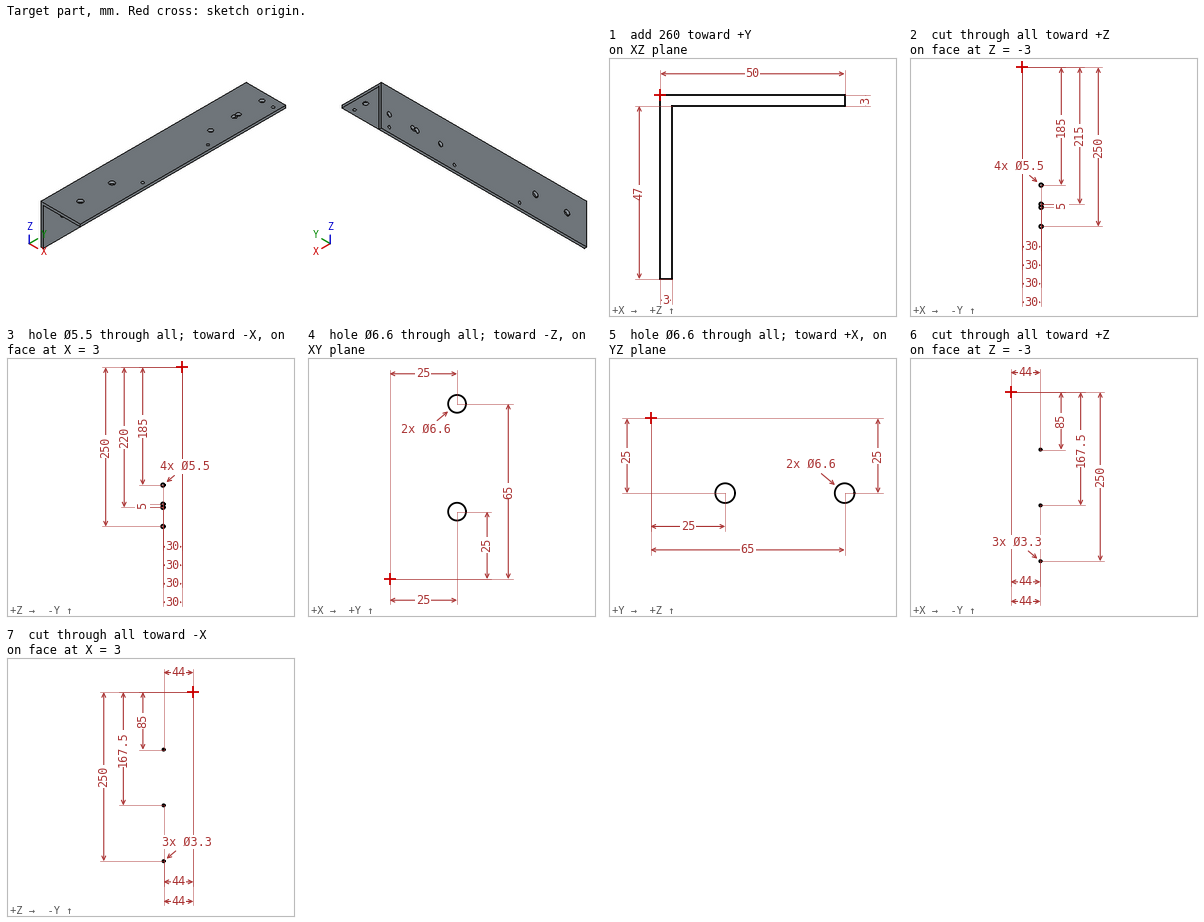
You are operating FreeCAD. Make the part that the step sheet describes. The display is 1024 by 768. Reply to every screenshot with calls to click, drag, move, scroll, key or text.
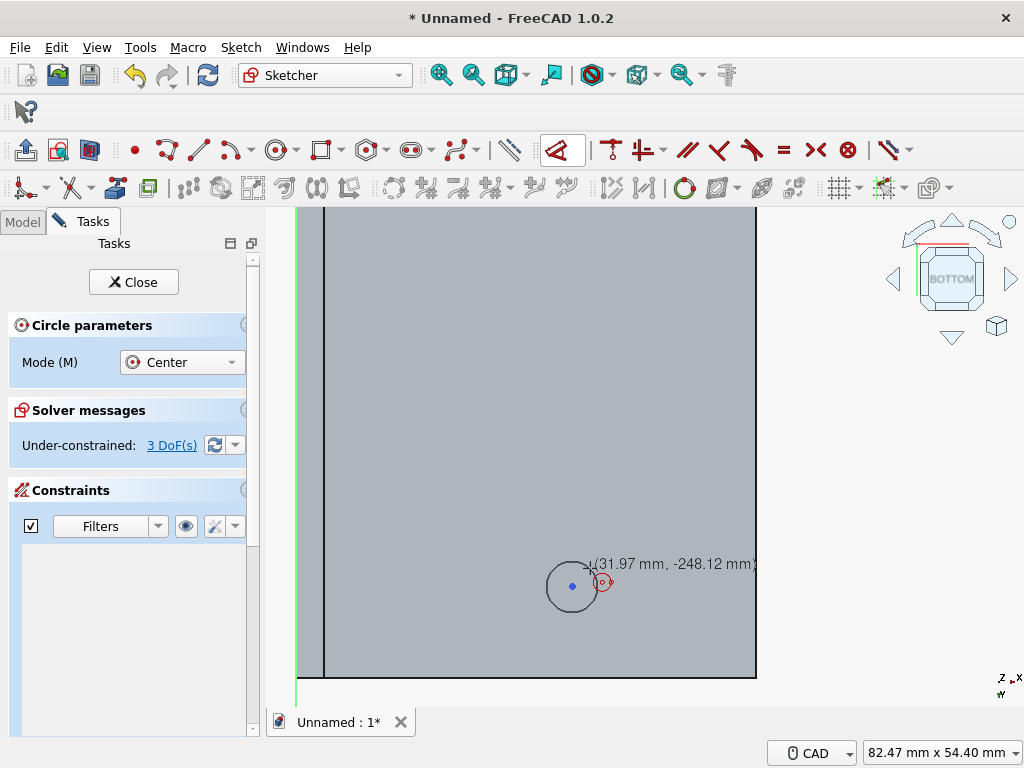
click(572, 265)
click(590, 247)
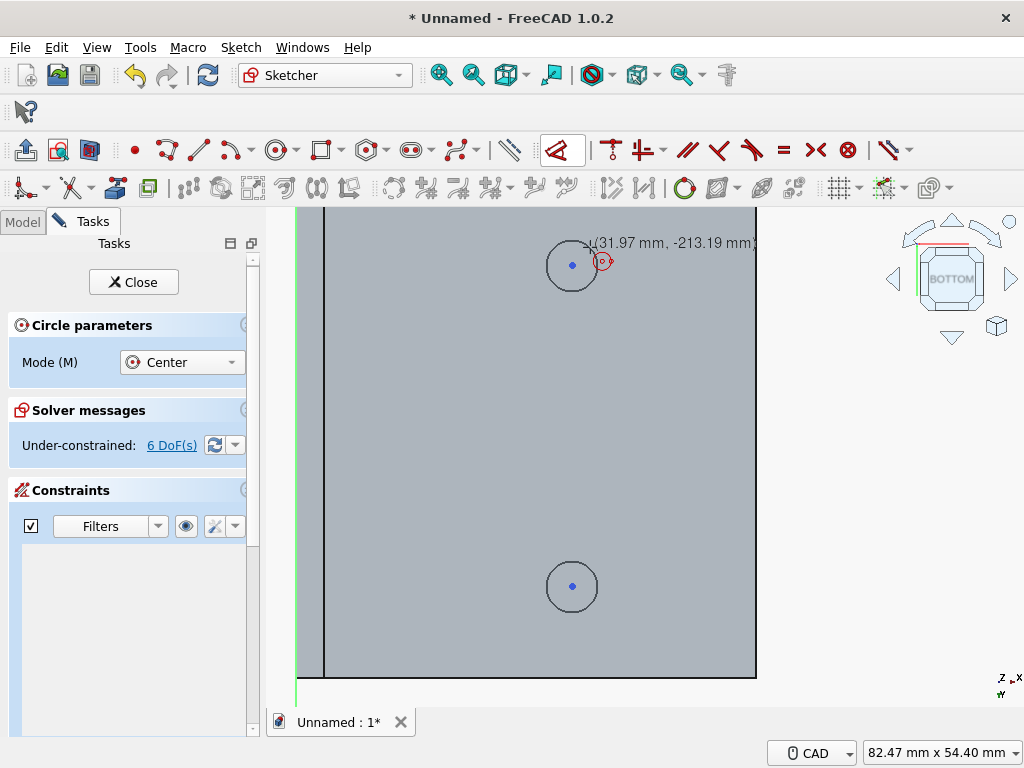
click(572, 311)
click(590, 328)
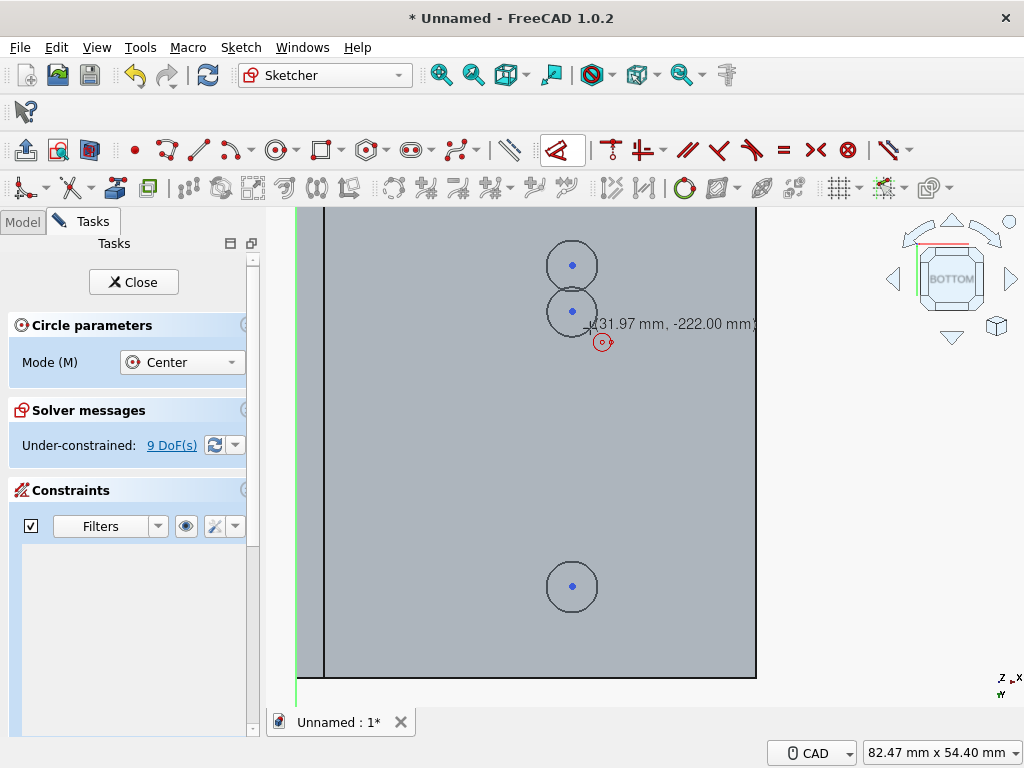
scroll(580, 595, down, 4)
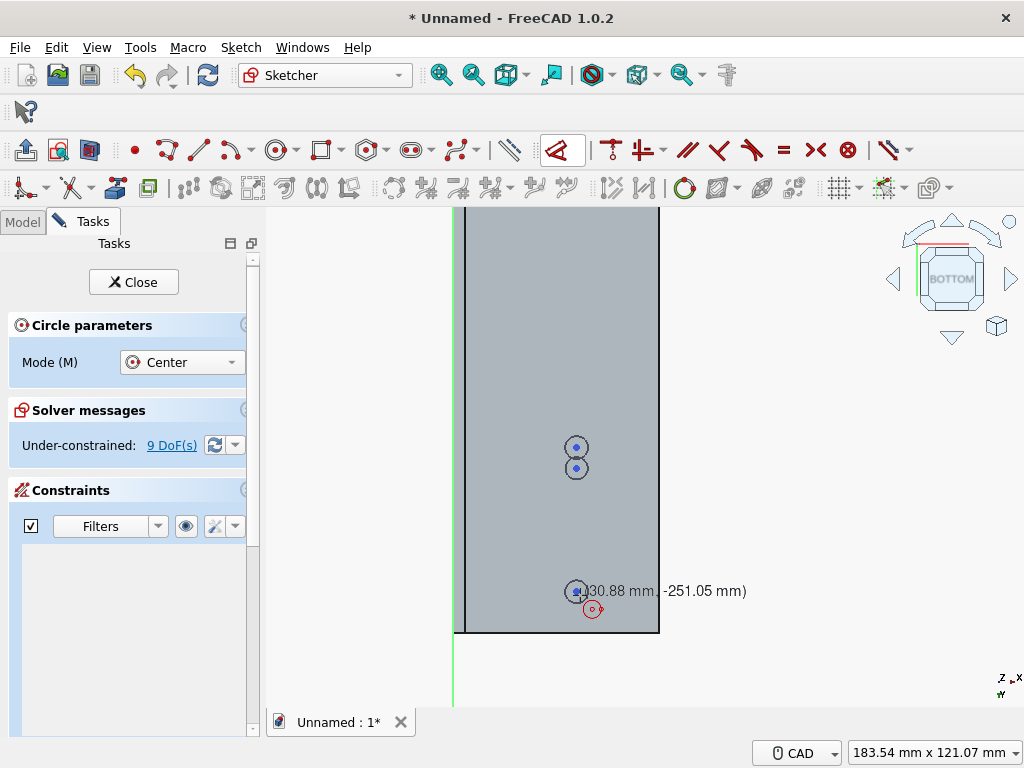
scroll(577, 323, up, 4)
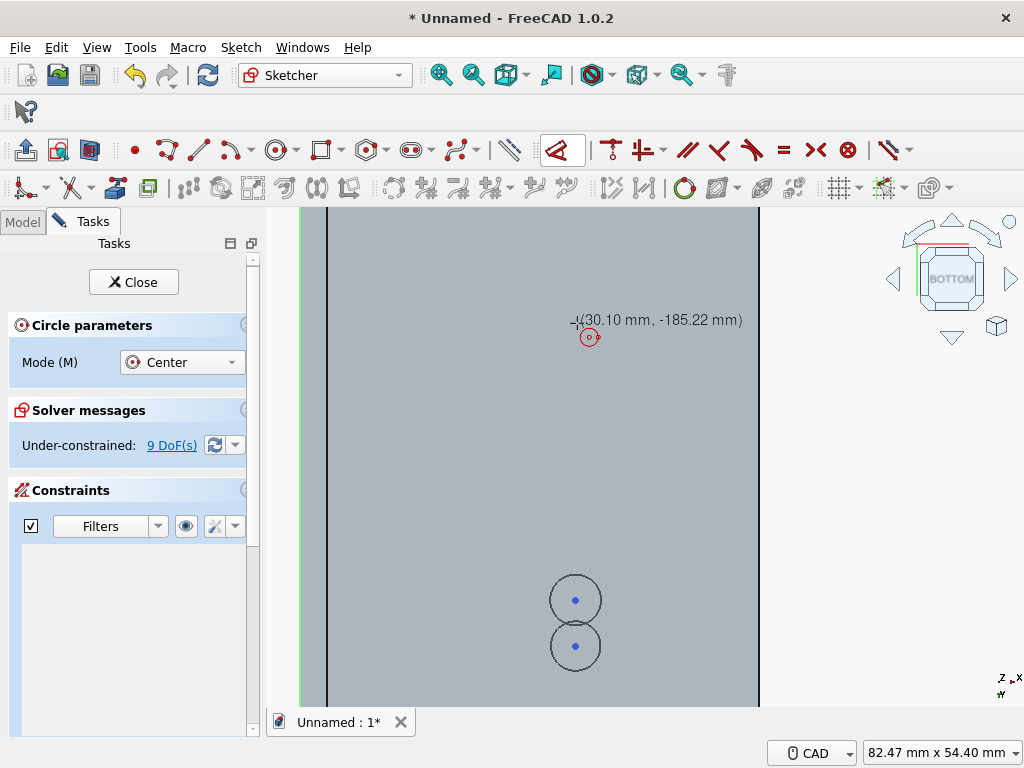
click(576, 323)
click(593, 305)
key(Escape)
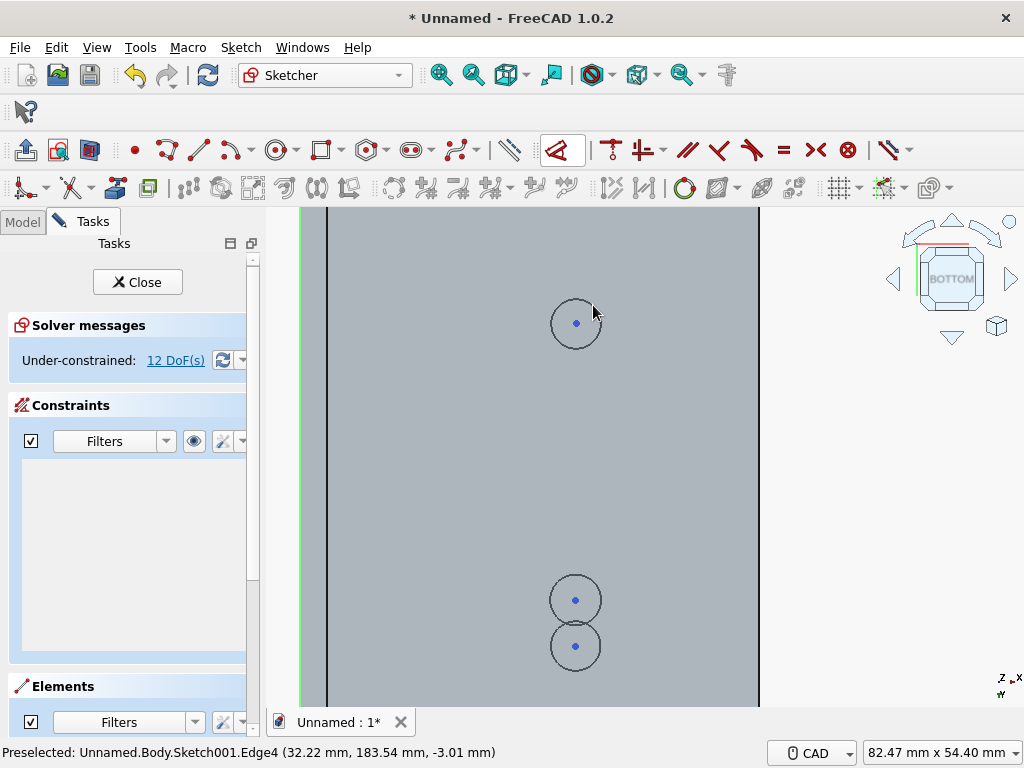
scroll(577, 323, down, 4)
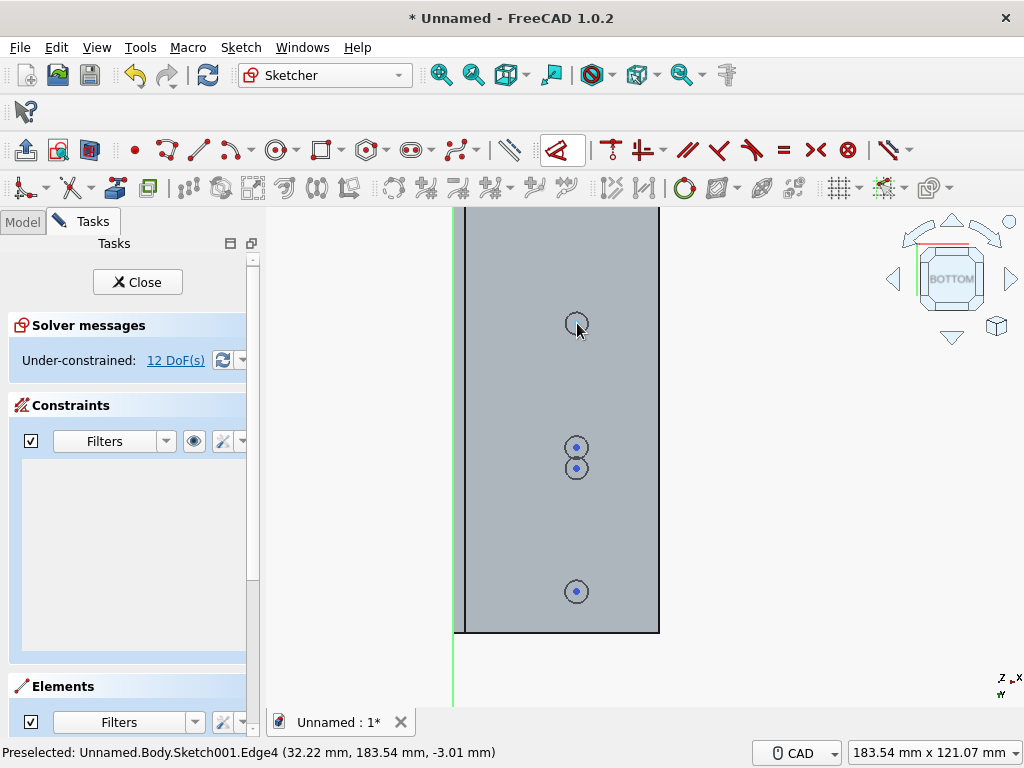
click(585, 584)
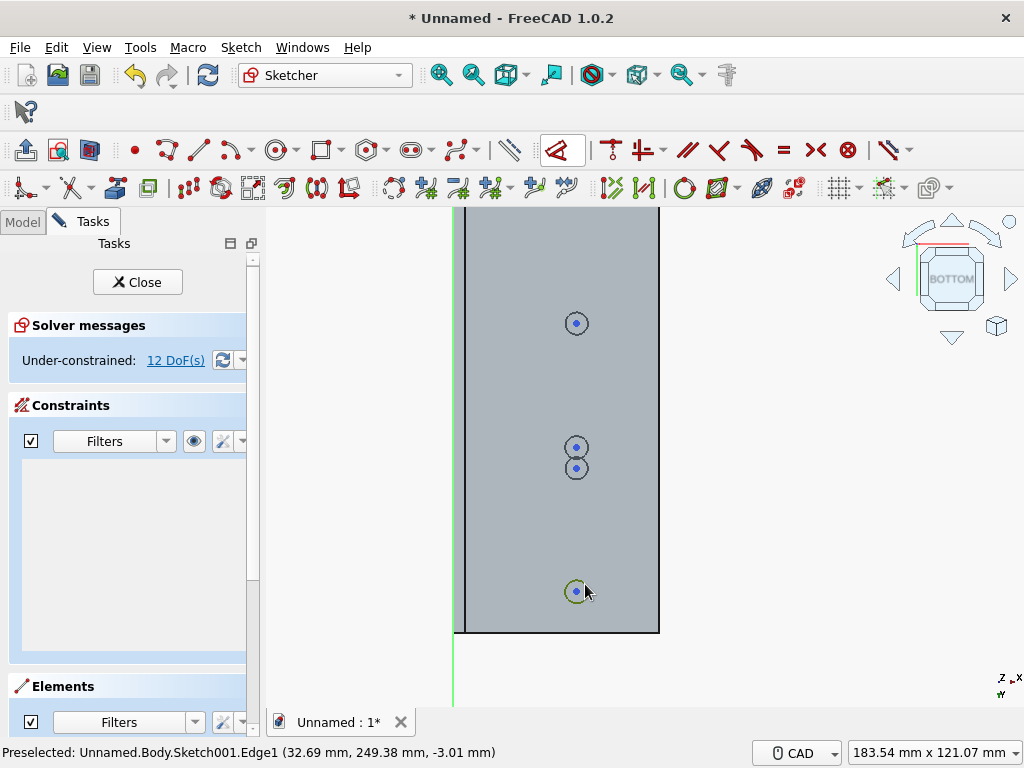
click(585, 439)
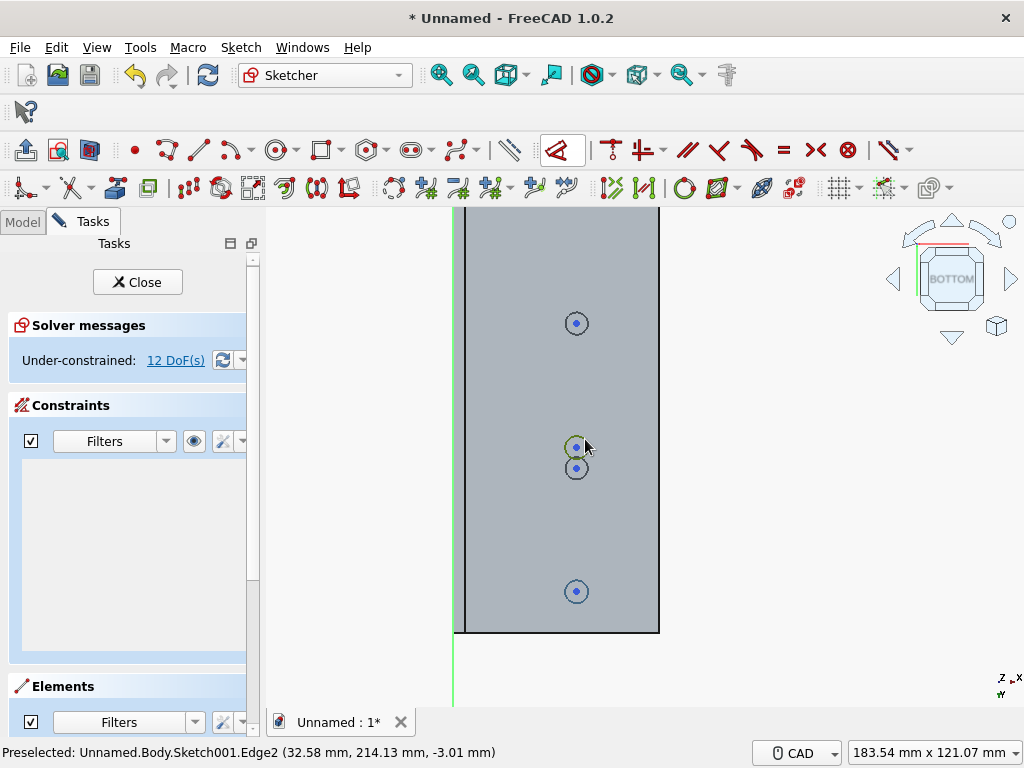
scroll(569, 476, up, 2)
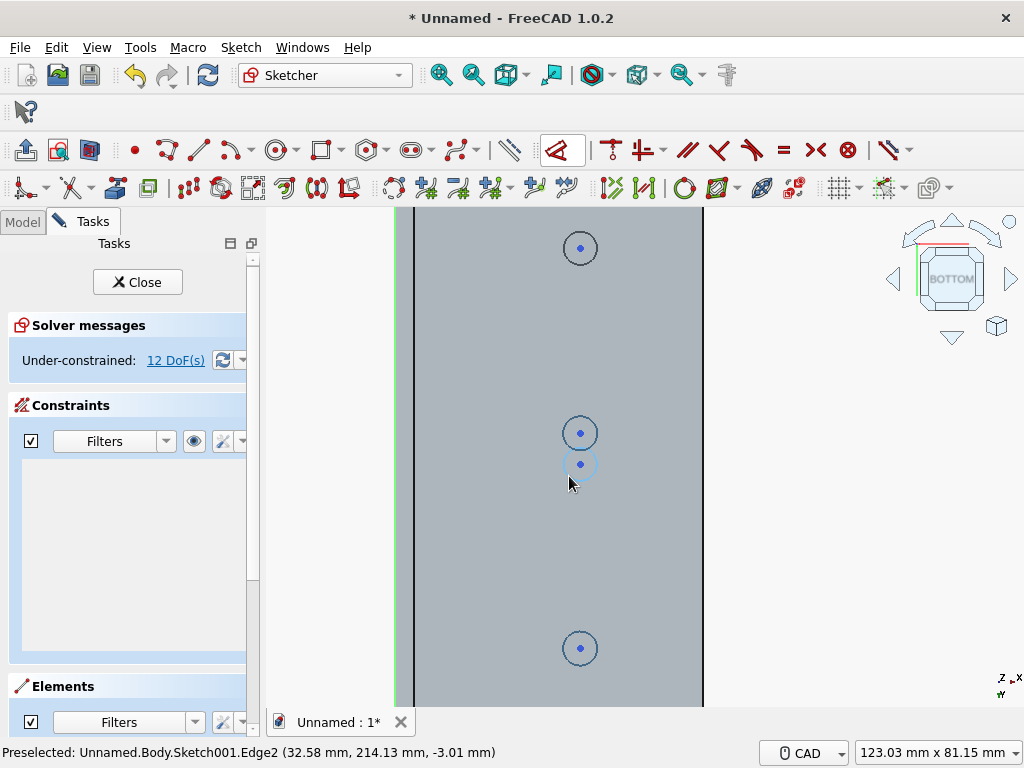
click(568, 476)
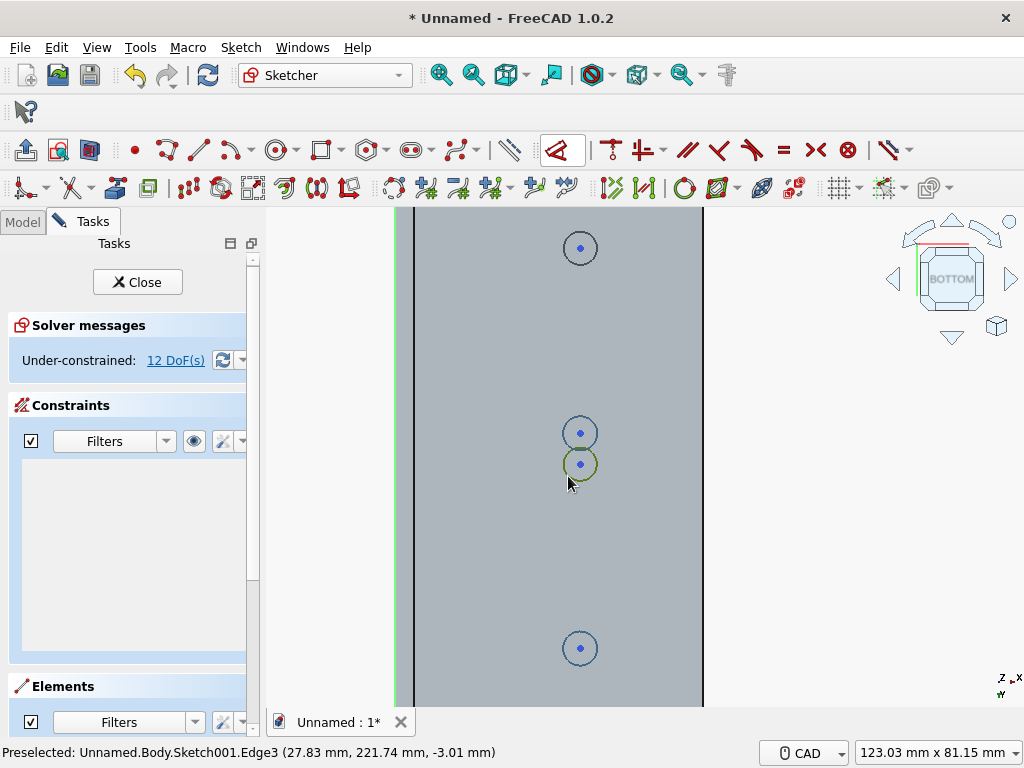
click(592, 237)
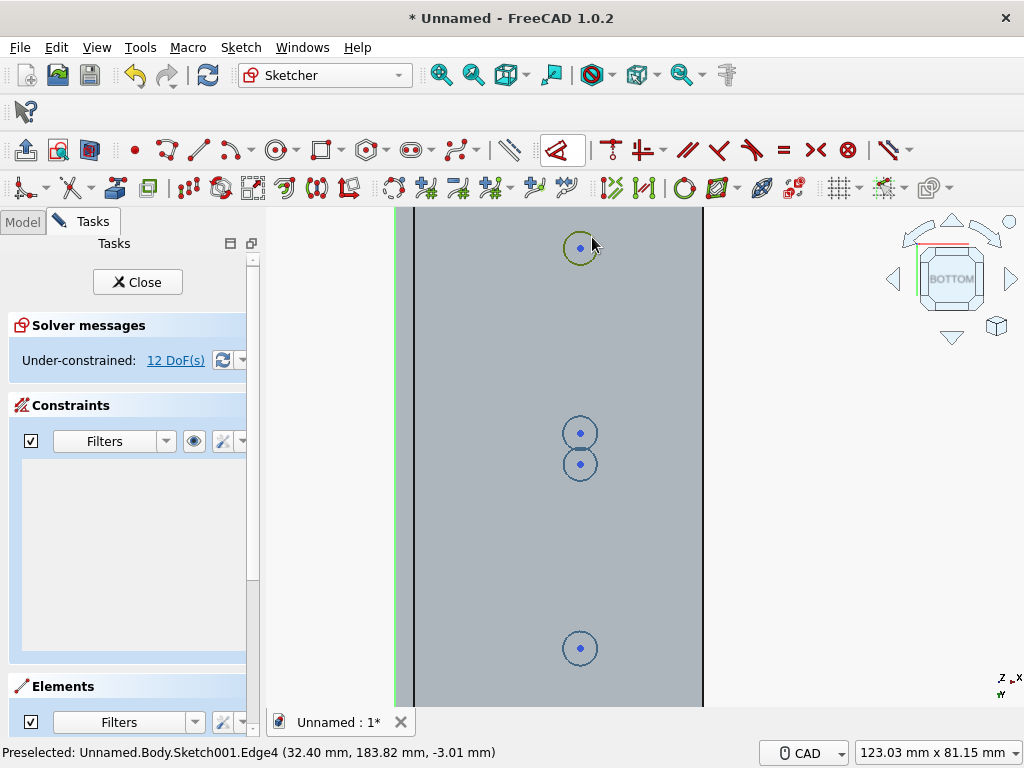
click(784, 150)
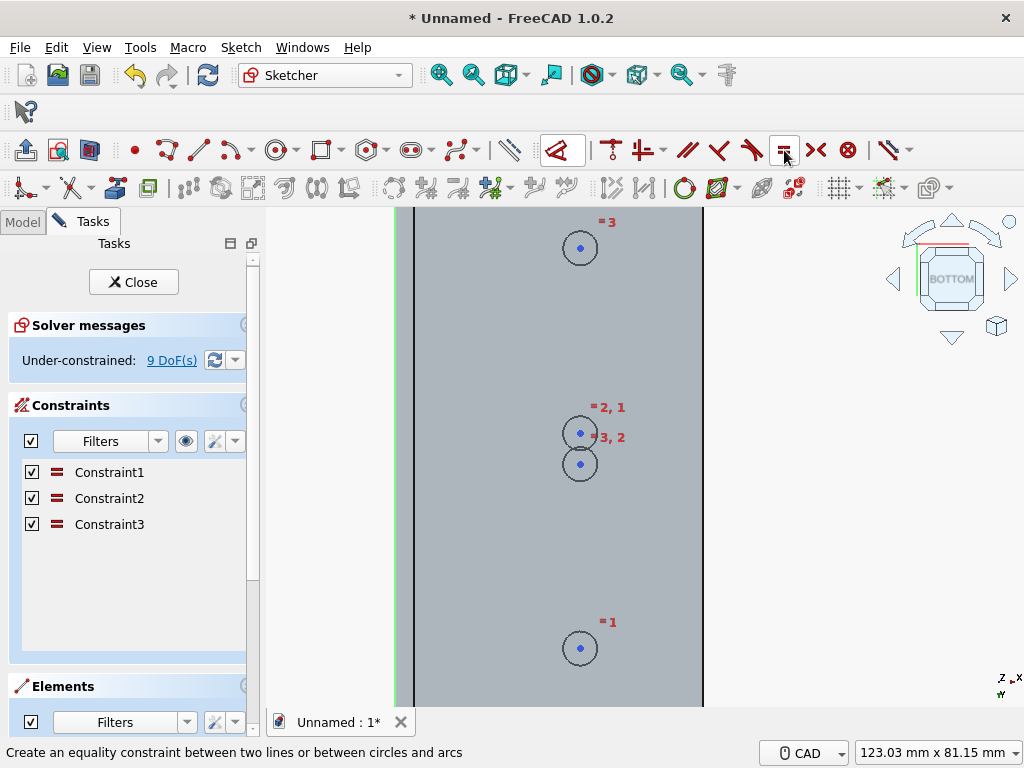
click(592, 636)